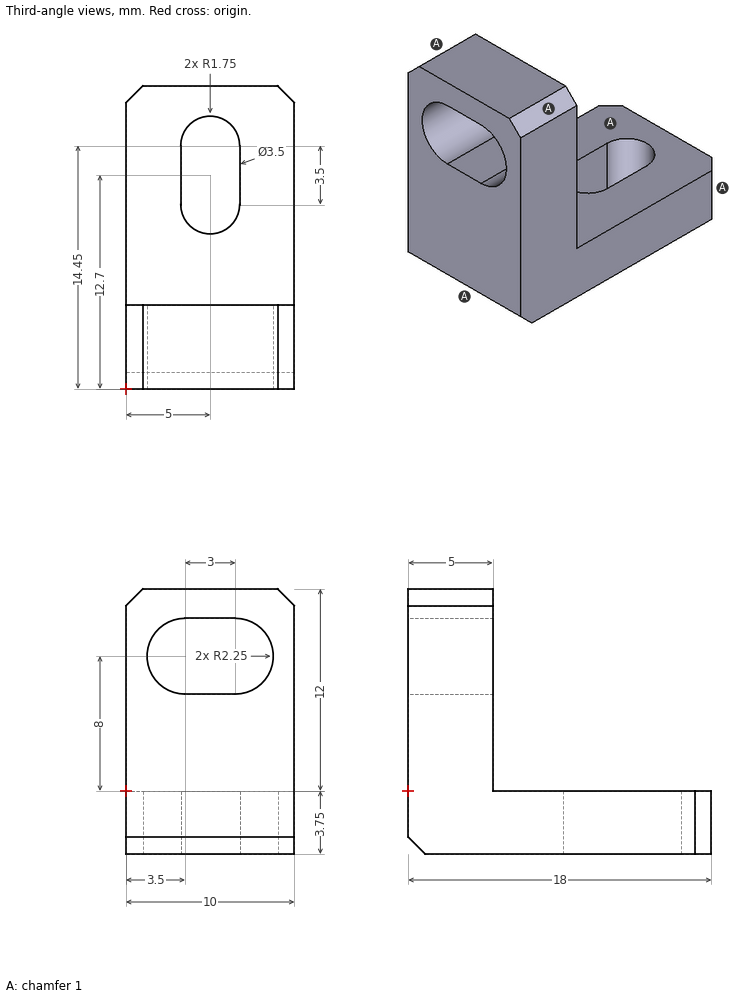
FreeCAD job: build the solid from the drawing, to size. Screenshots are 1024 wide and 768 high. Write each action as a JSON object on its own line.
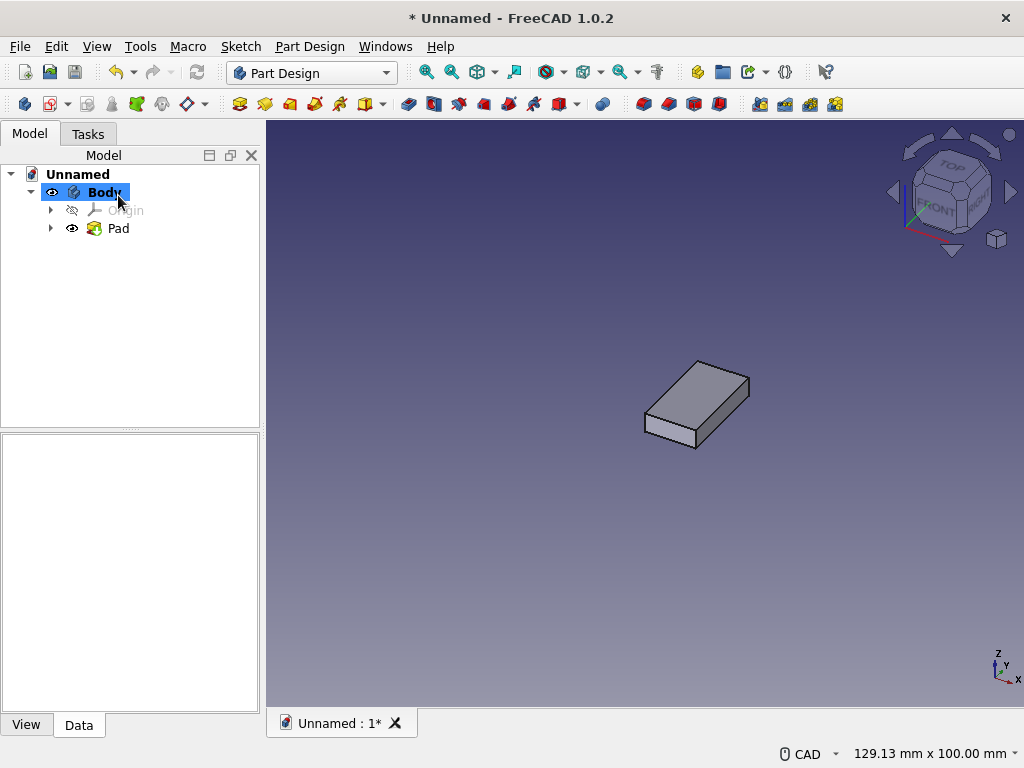
{"action": "left_click", "coordinate": [427, 72]}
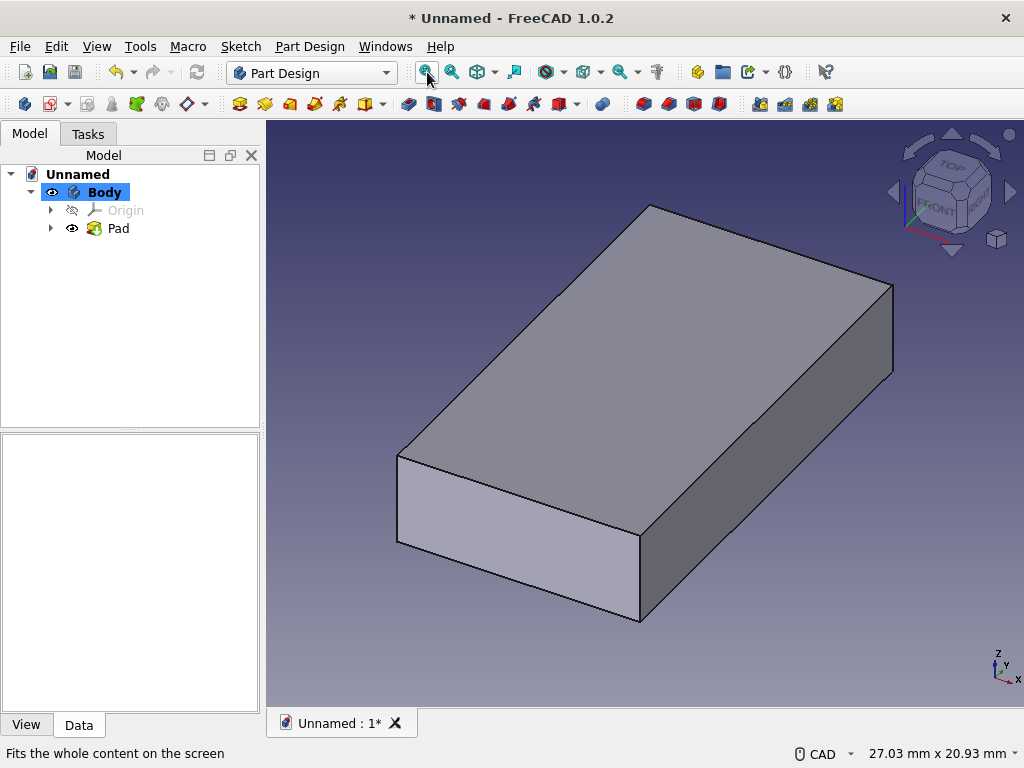
{"action": "left_click", "coordinate": [50, 104]}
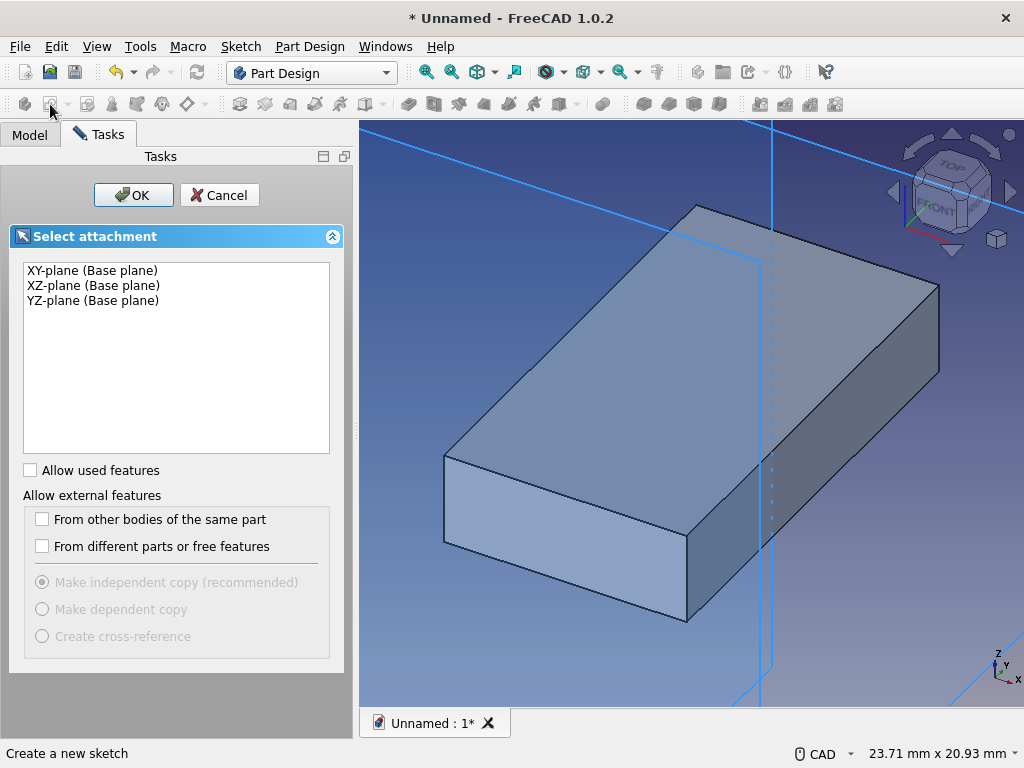
{"action": "left_click", "coordinate": [84, 270]}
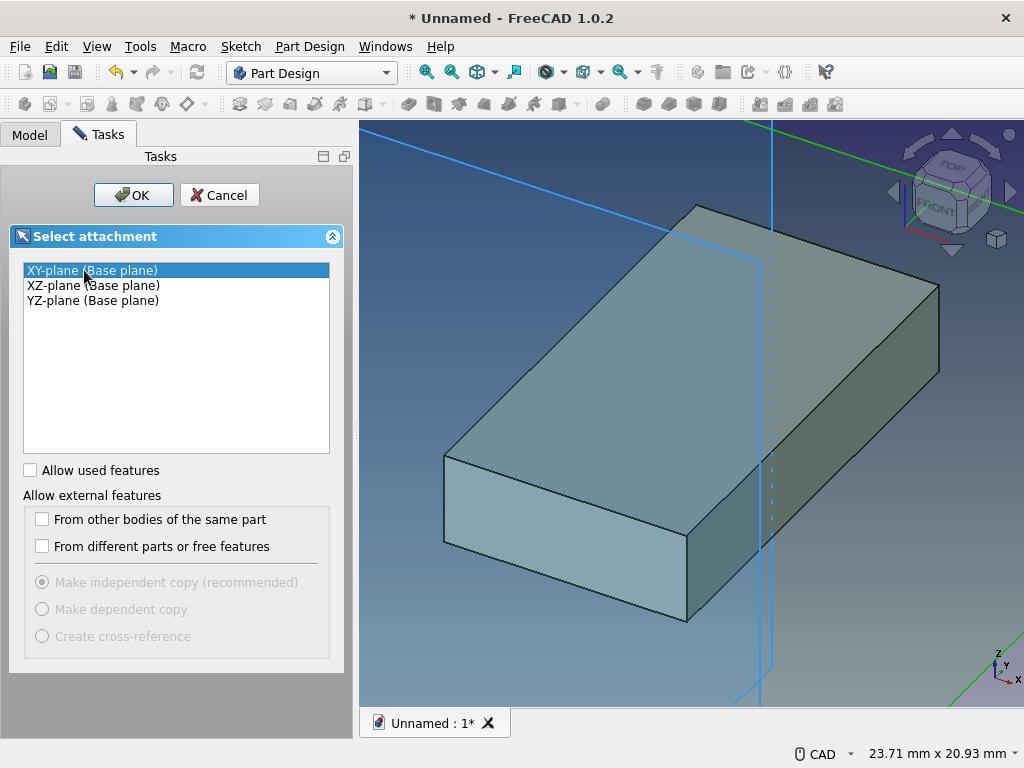
{"action": "left_click", "coordinate": [134, 195]}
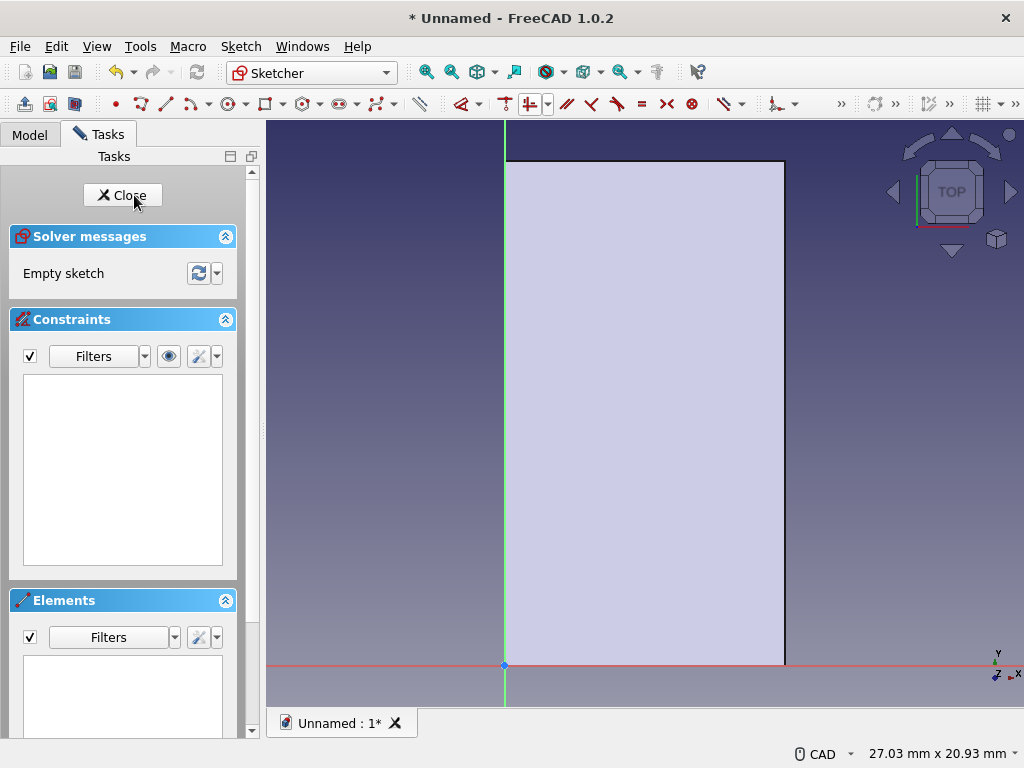
{"action": "scroll", "coordinate": [667, 276], "scroll_direction": "up", "scroll_amount": 7}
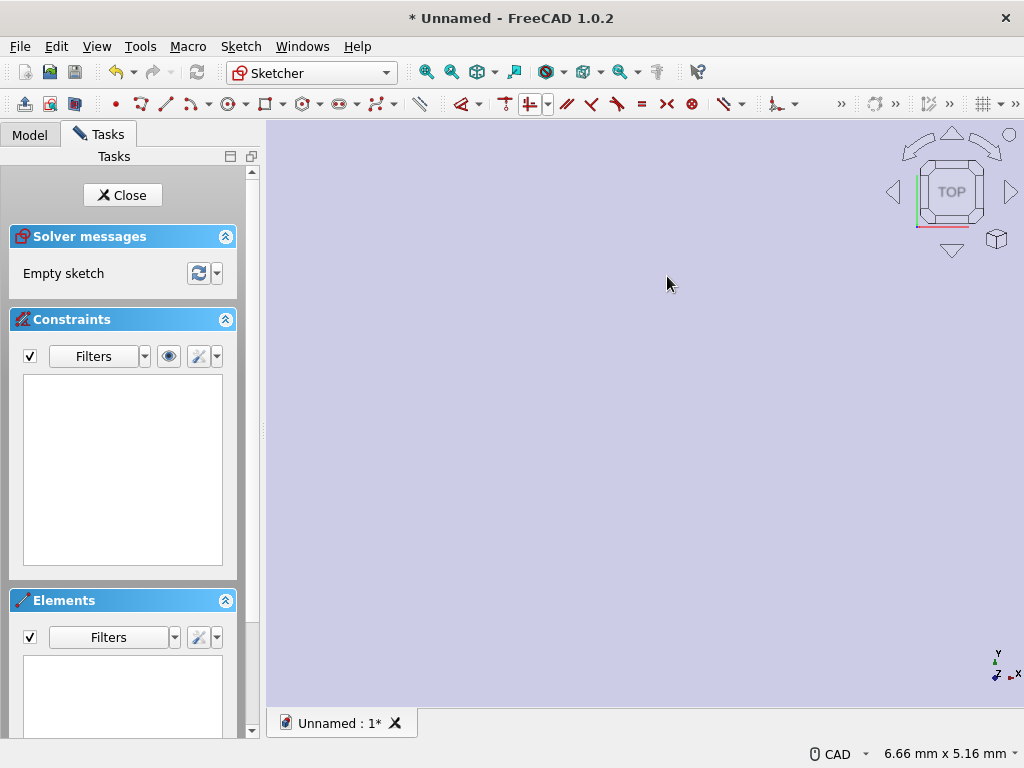
{"action": "left_click", "coordinate": [228, 104]}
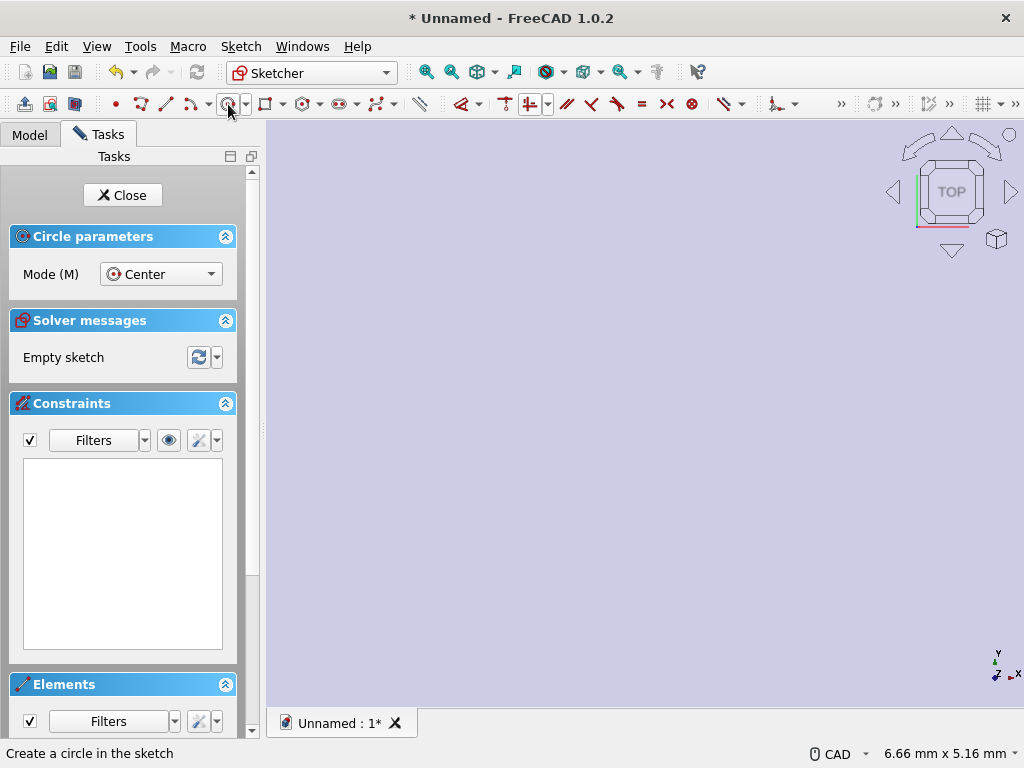
{"action": "left_click", "coordinate": [576, 412]}
{"action": "mouse_move", "coordinate": [717, 271]}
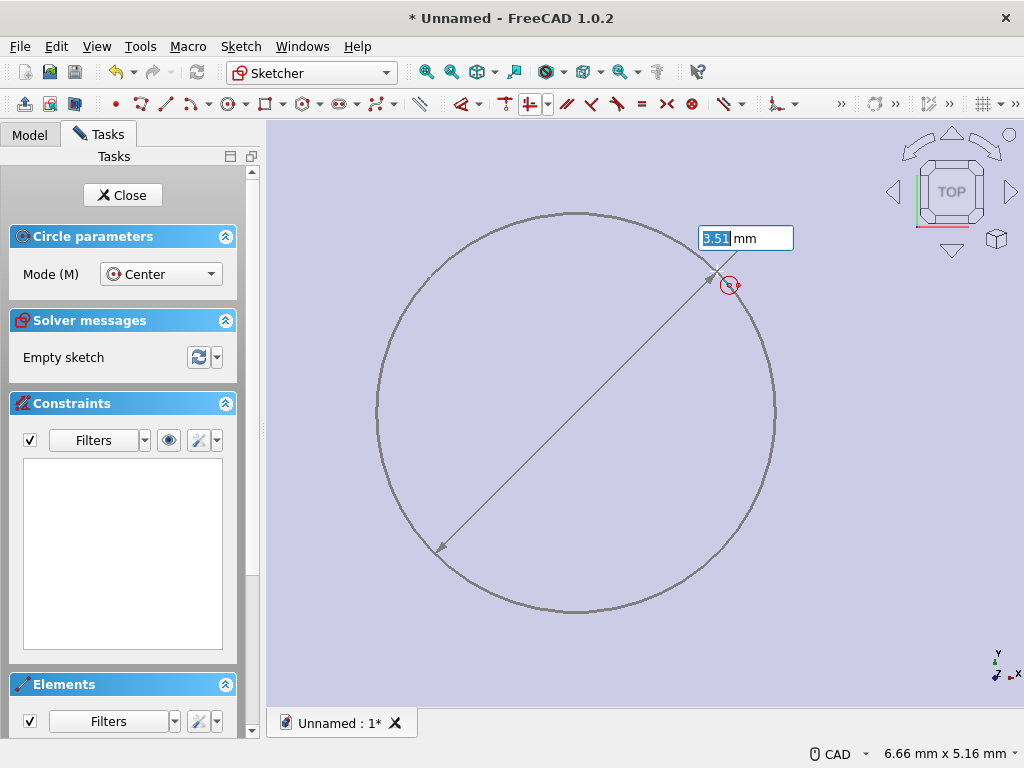
{"action": "type", "text": "3.5"}
{"action": "key", "text": "Return"}
{"action": "key", "text": "Escape"}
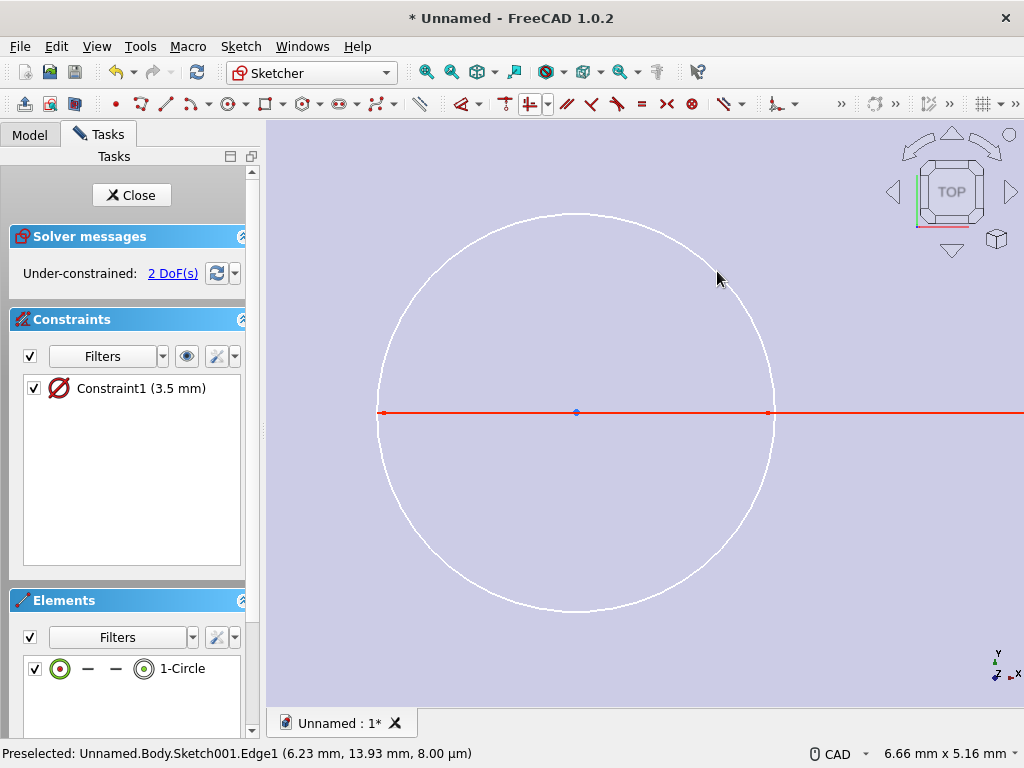
{"action": "left_click", "coordinate": [460, 104]}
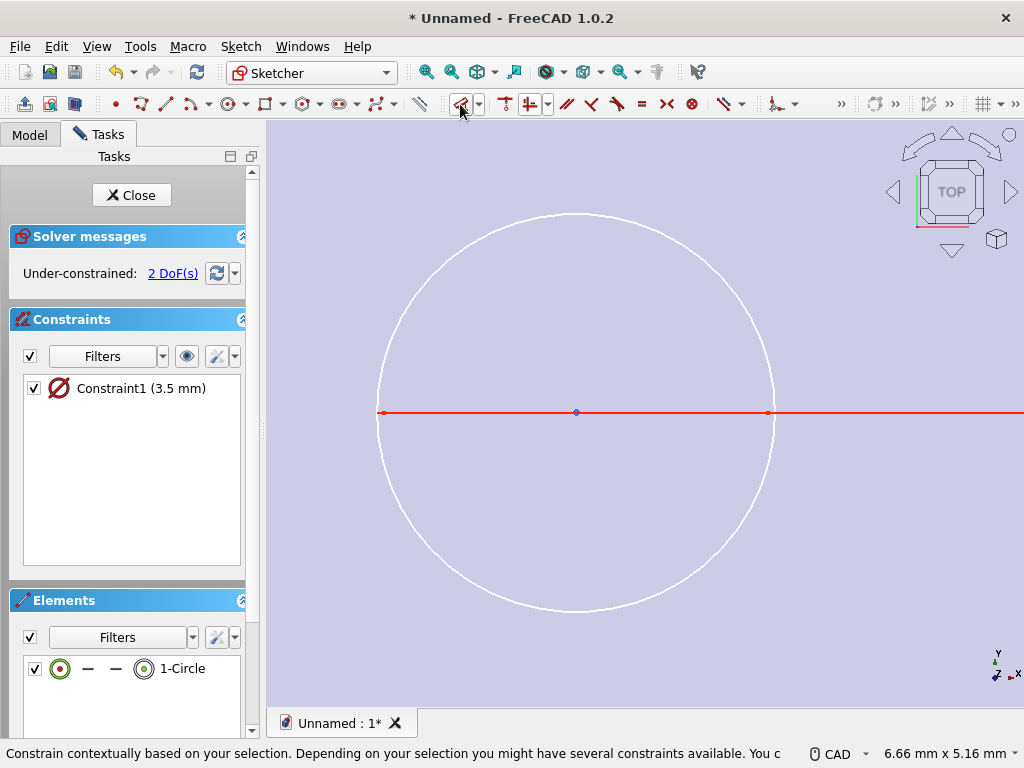
{"action": "left_click", "coordinate": [576, 413]}
{"action": "left_click", "coordinate": [435, 379]}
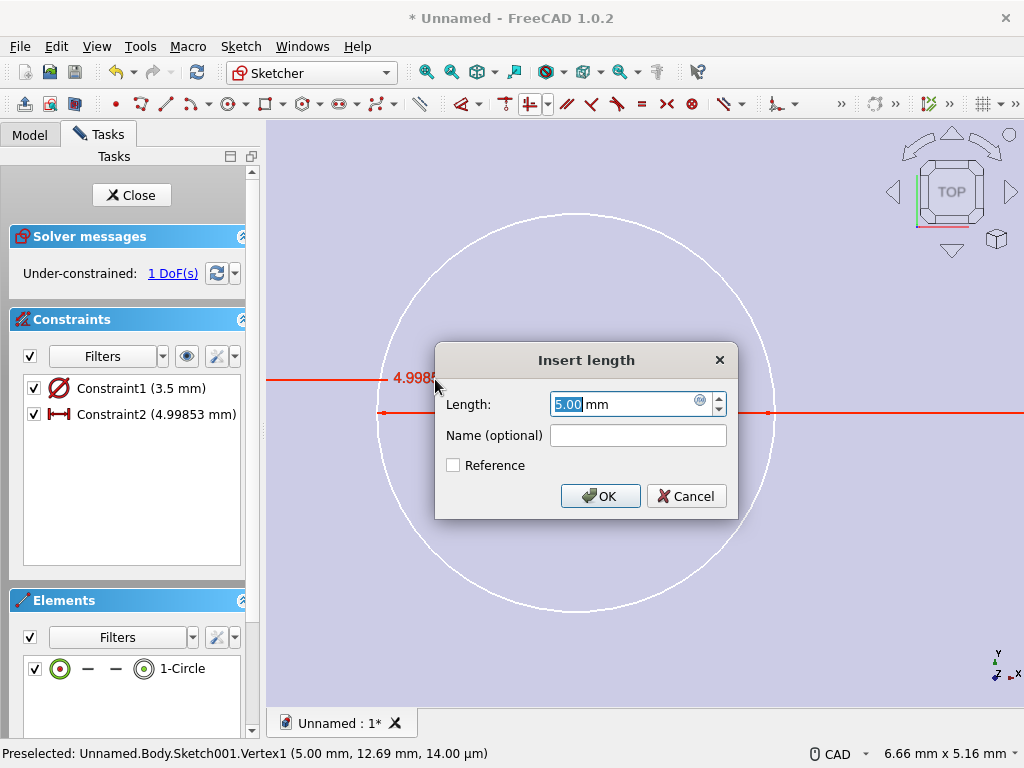
{"action": "type", "text": "5"}
{"action": "key", "text": "Return"}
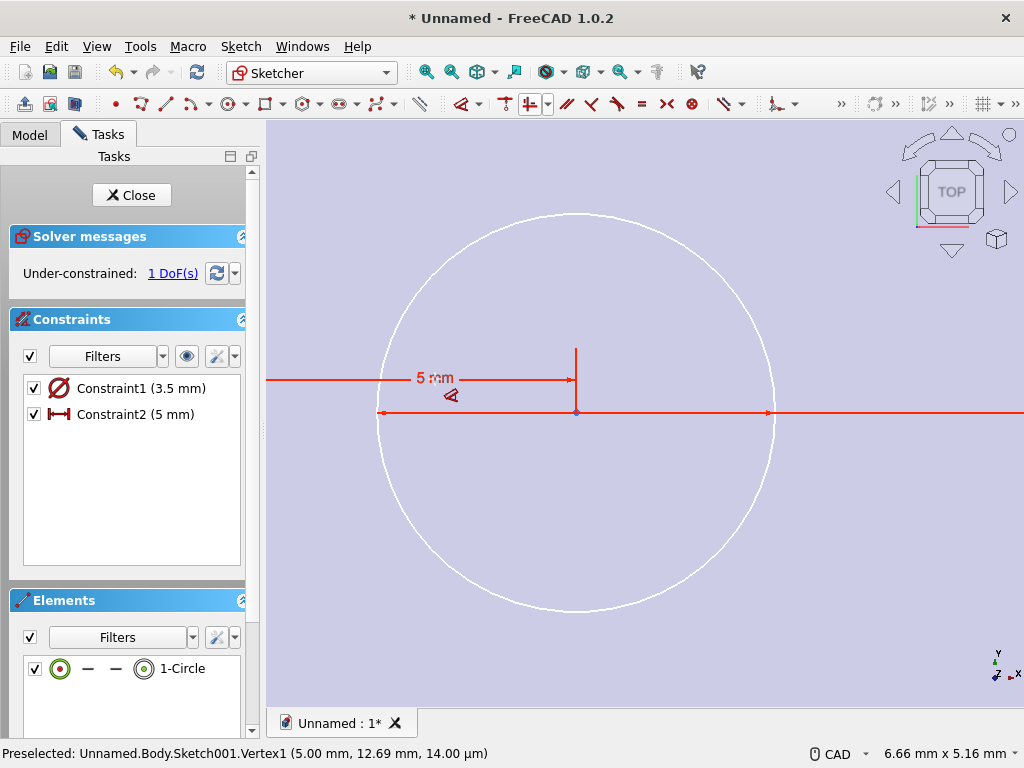
{"action": "left_click", "coordinate": [576, 413]}
{"action": "left_click", "coordinate": [610, 546]}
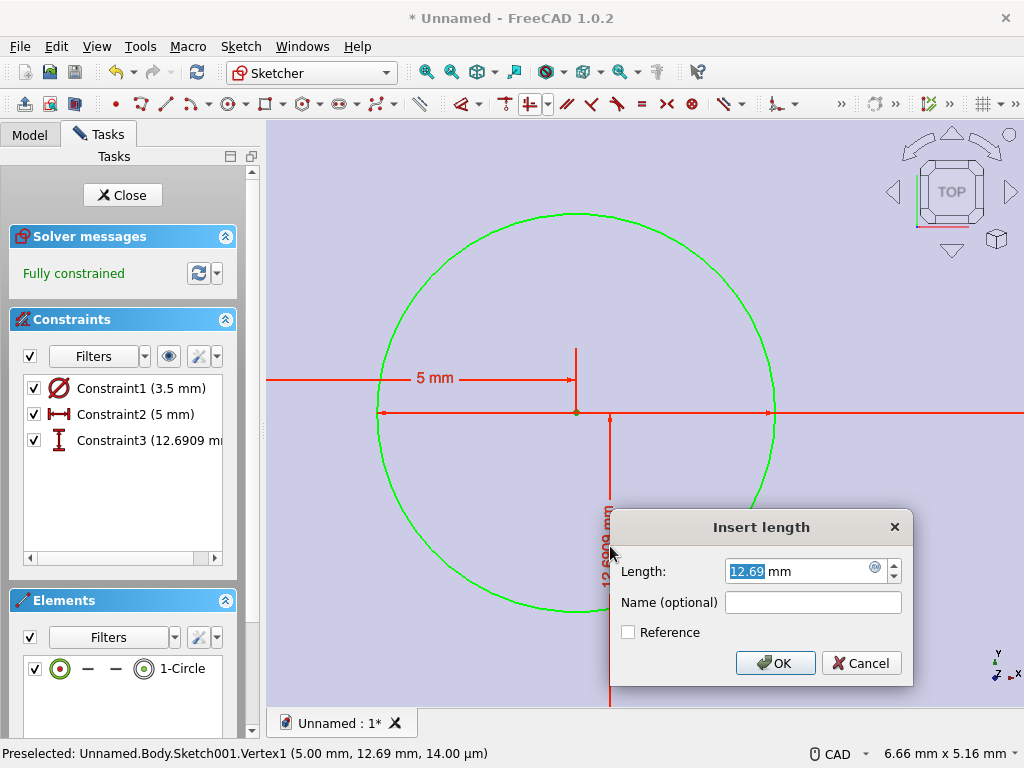
{"action": "type", "text": "12.7"}
{"action": "key", "text": "Return"}
{"action": "key", "text": "Escape"}